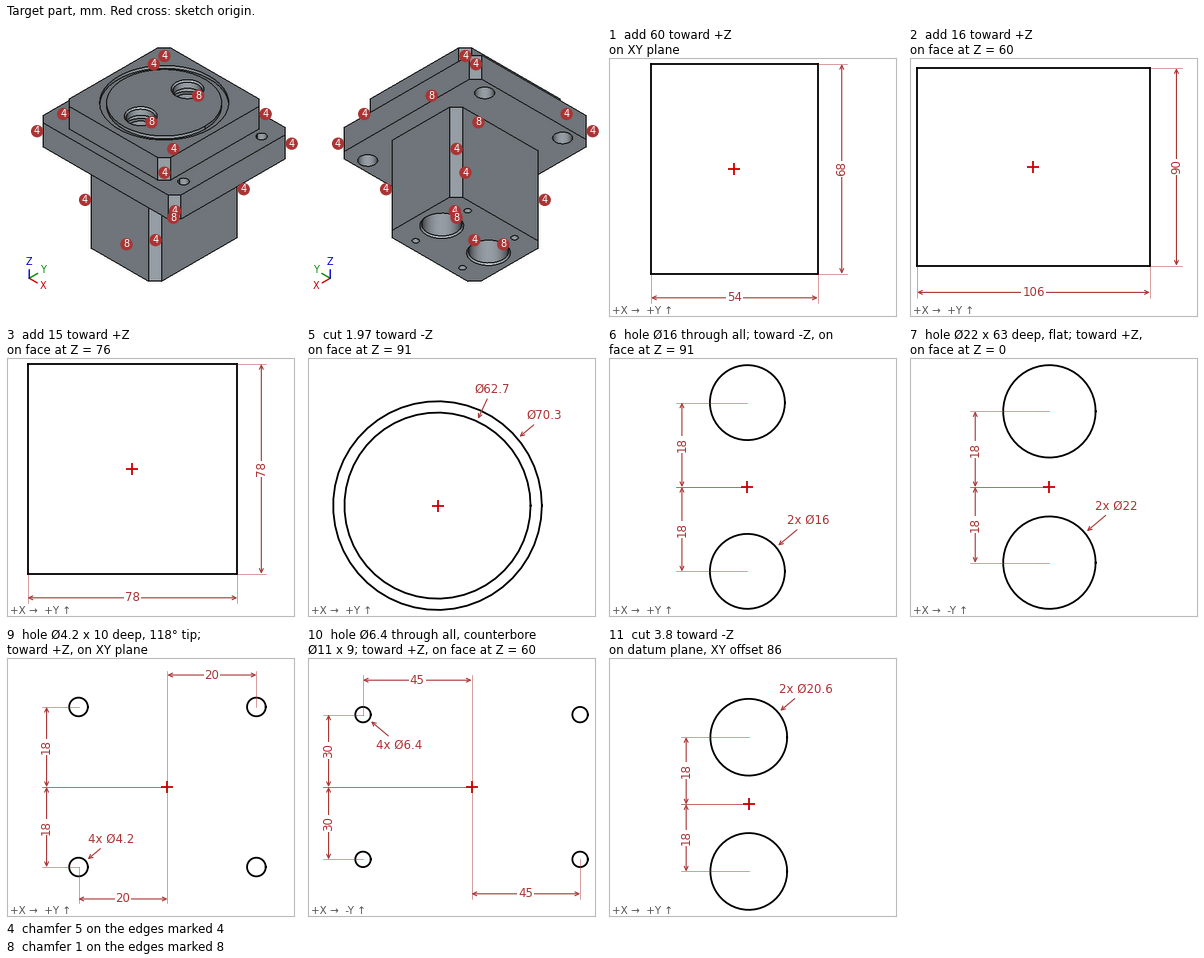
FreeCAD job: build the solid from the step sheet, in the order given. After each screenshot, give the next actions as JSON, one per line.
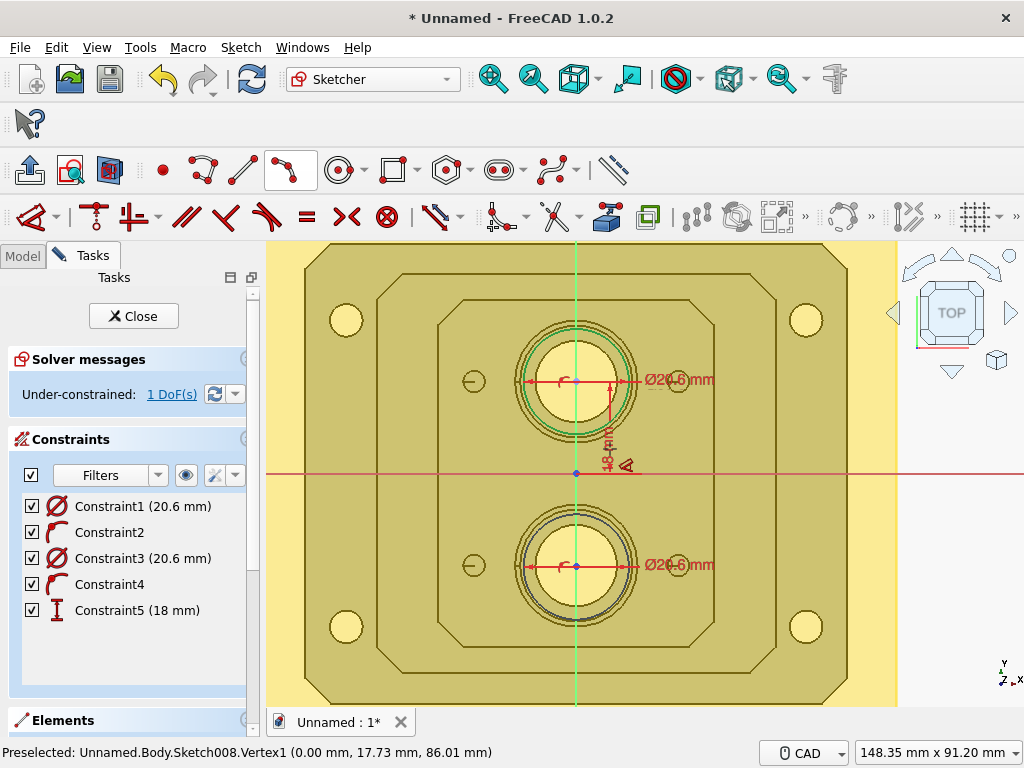
{"action": "left_click", "coordinate": [576, 567]}
{"action": "left_click", "coordinate": [610, 499]}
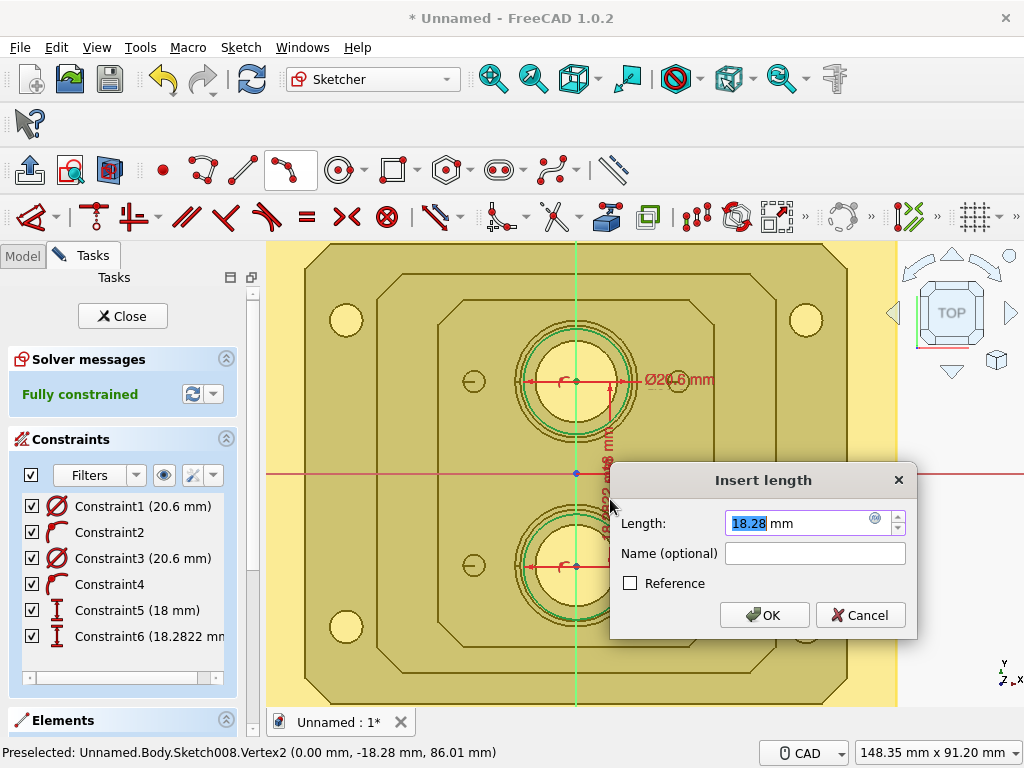
{"action": "type", "text": "18"}
{"action": "key", "text": "Return"}
{"action": "key", "text": "Escape"}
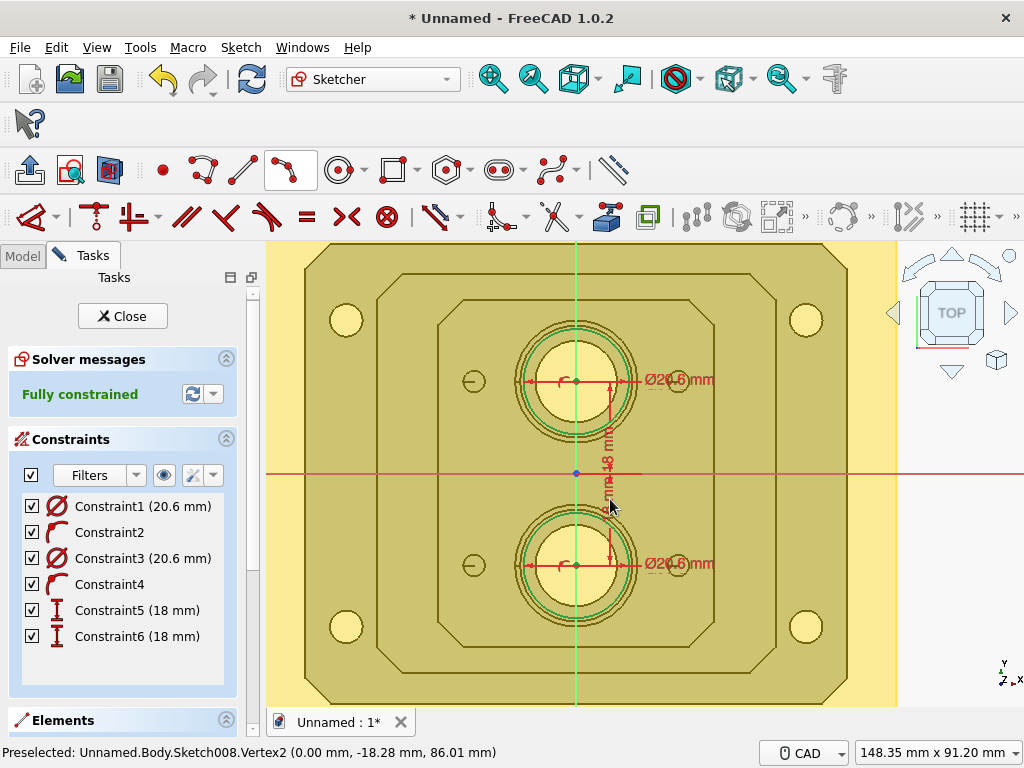
{"action": "left_click", "coordinate": [123, 316]}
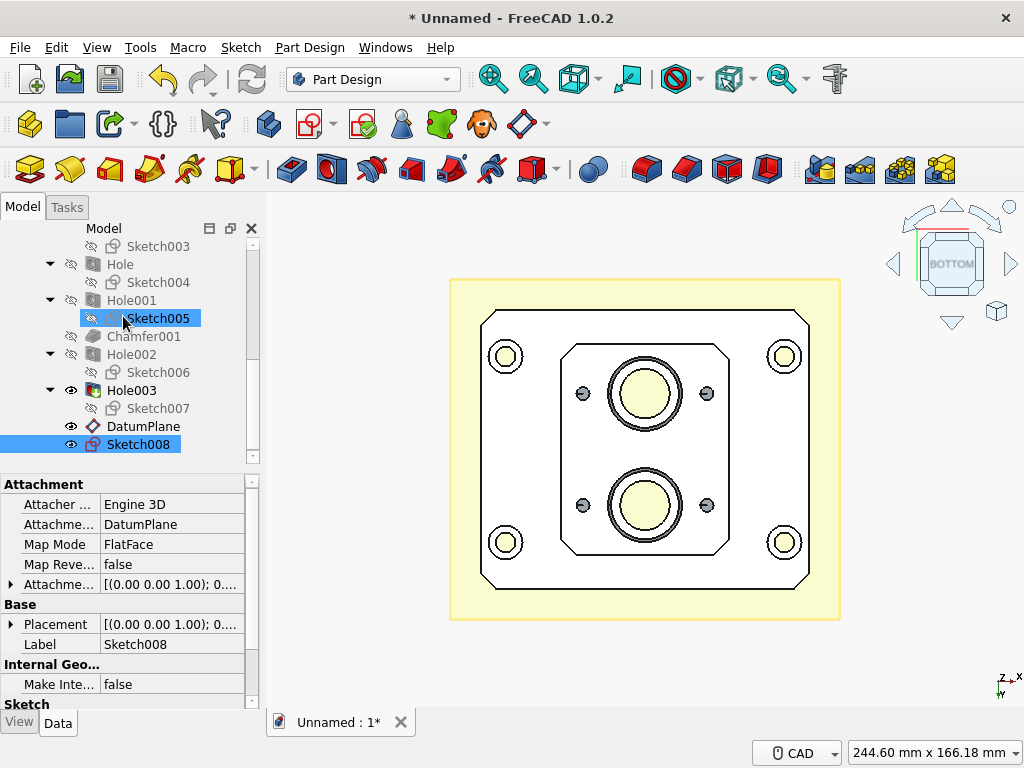
{"action": "left_click", "coordinate": [292, 170]}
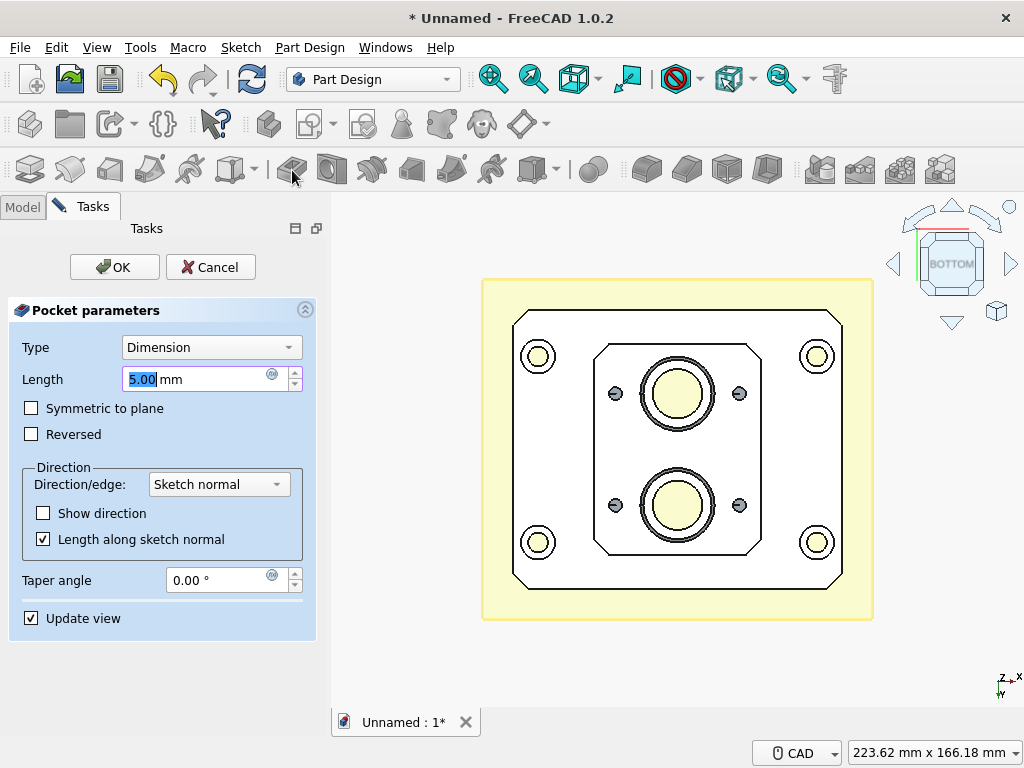
{"action": "type", "text": "3.8"}
{"action": "key", "text": "Tab"}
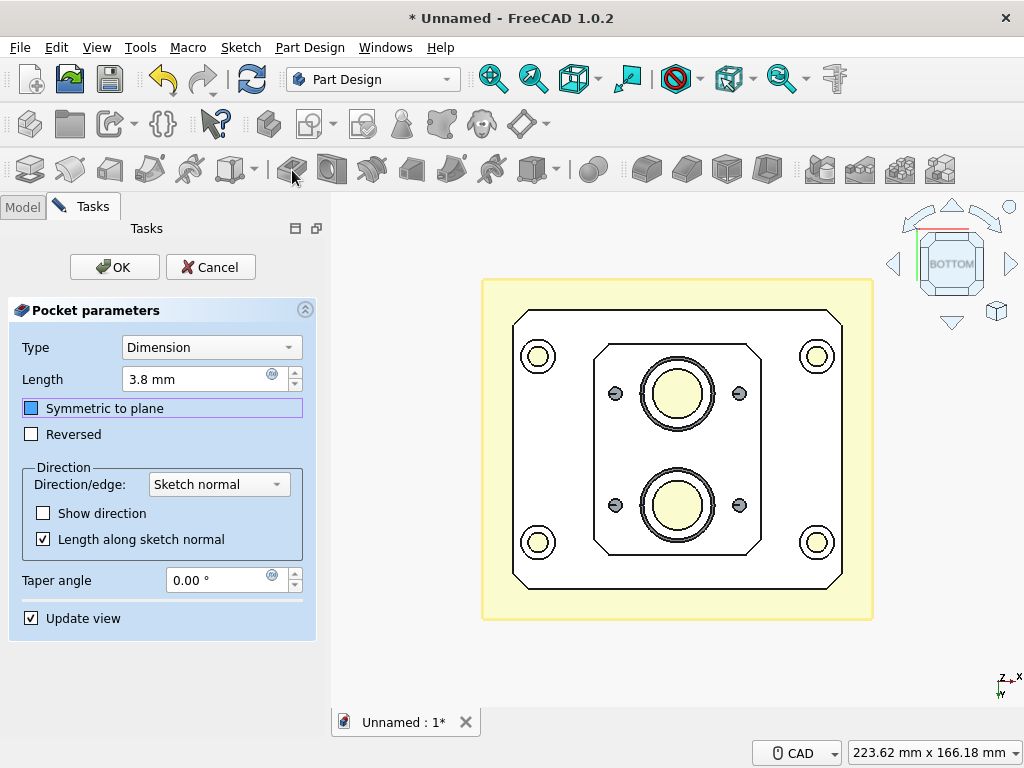
{"action": "left_click", "coordinate": [115, 267]}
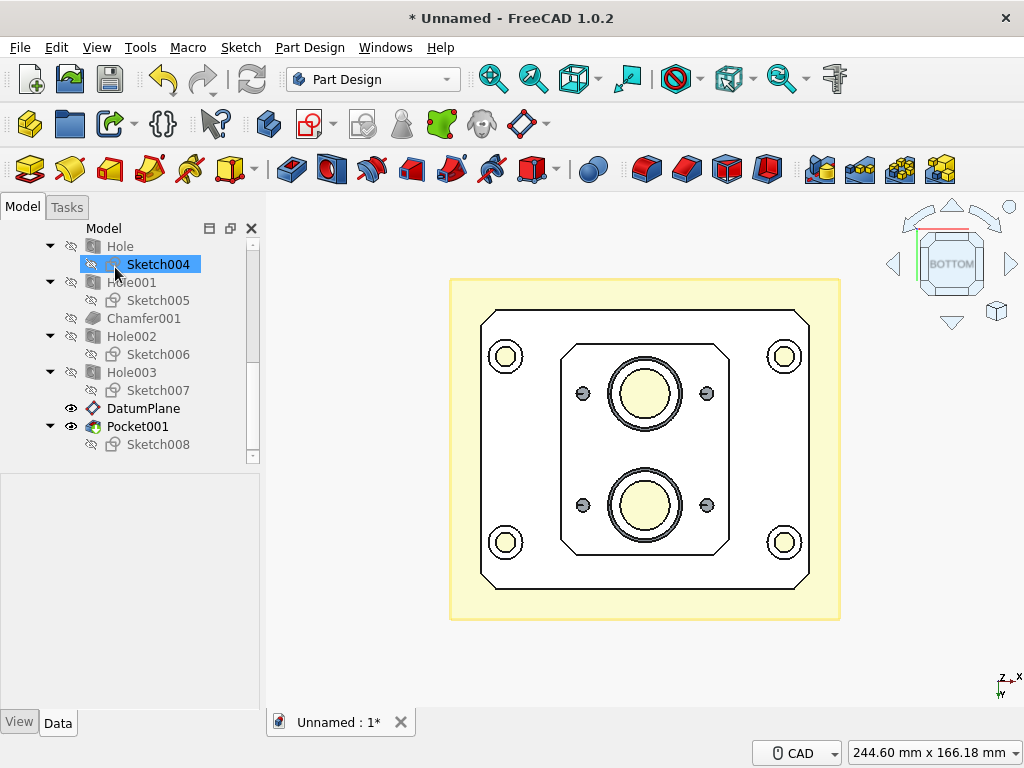
{"action": "left_click", "coordinate": [116, 408]}
{"action": "key", "text": "space"}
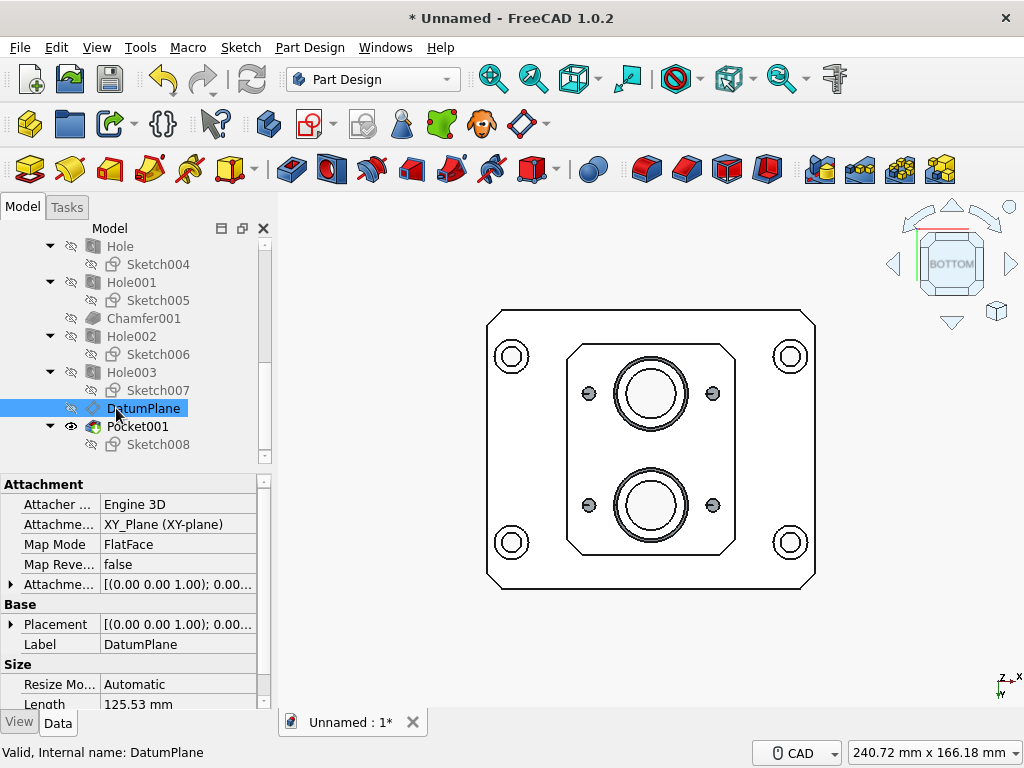
{"action": "key", "text": "0"}